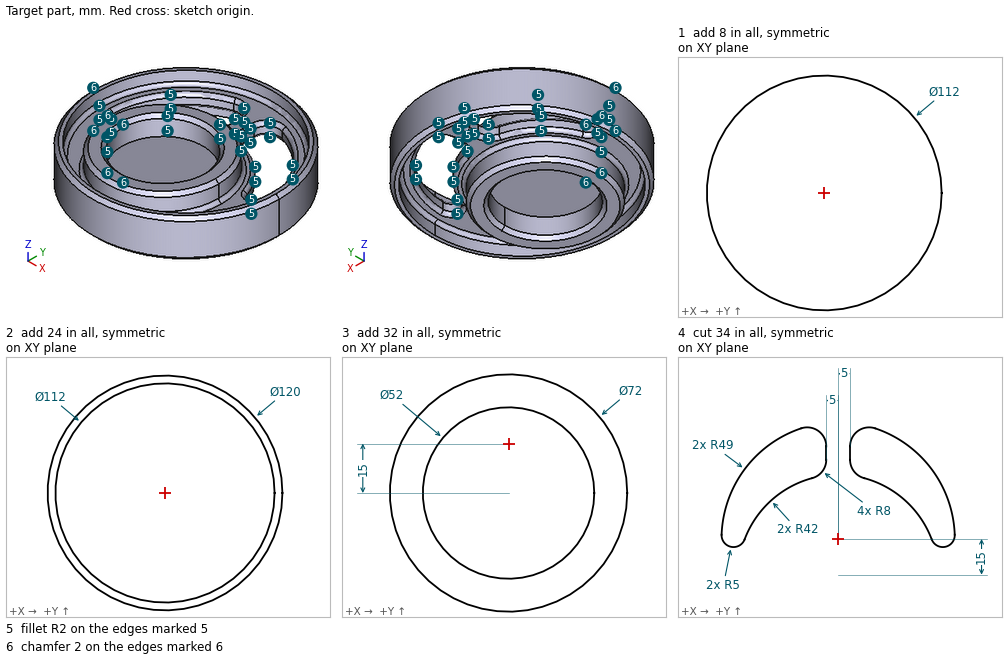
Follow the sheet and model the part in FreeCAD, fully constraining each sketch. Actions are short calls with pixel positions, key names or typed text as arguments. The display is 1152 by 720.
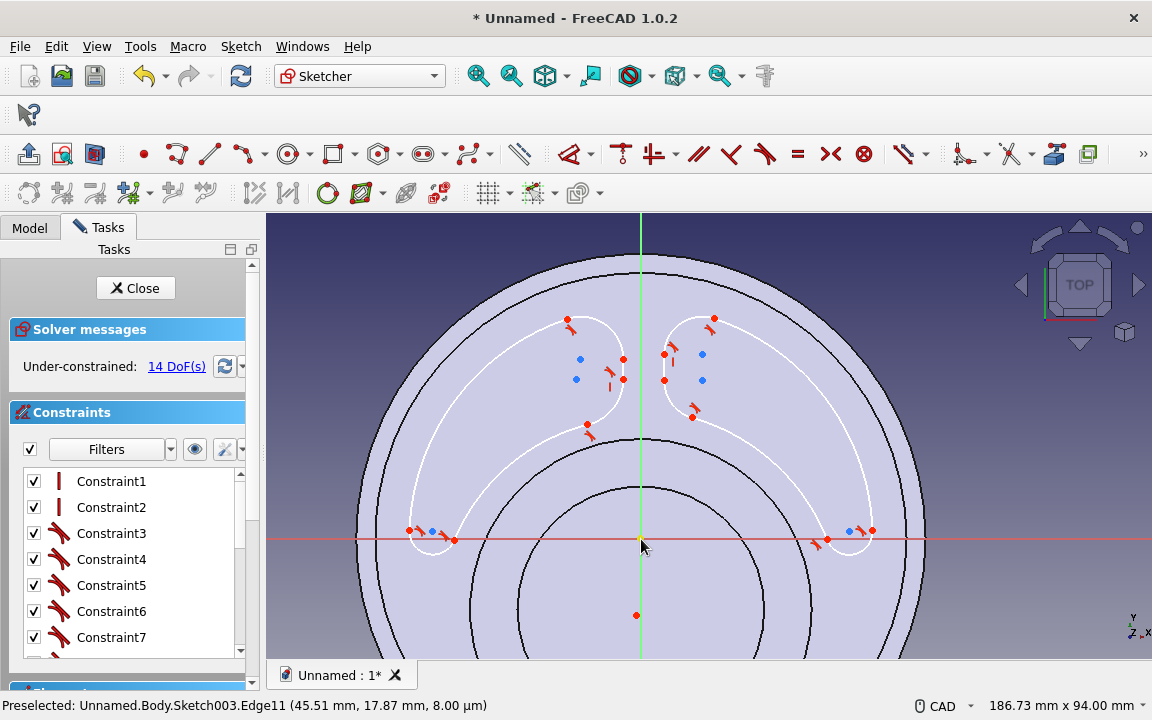
click(617, 336)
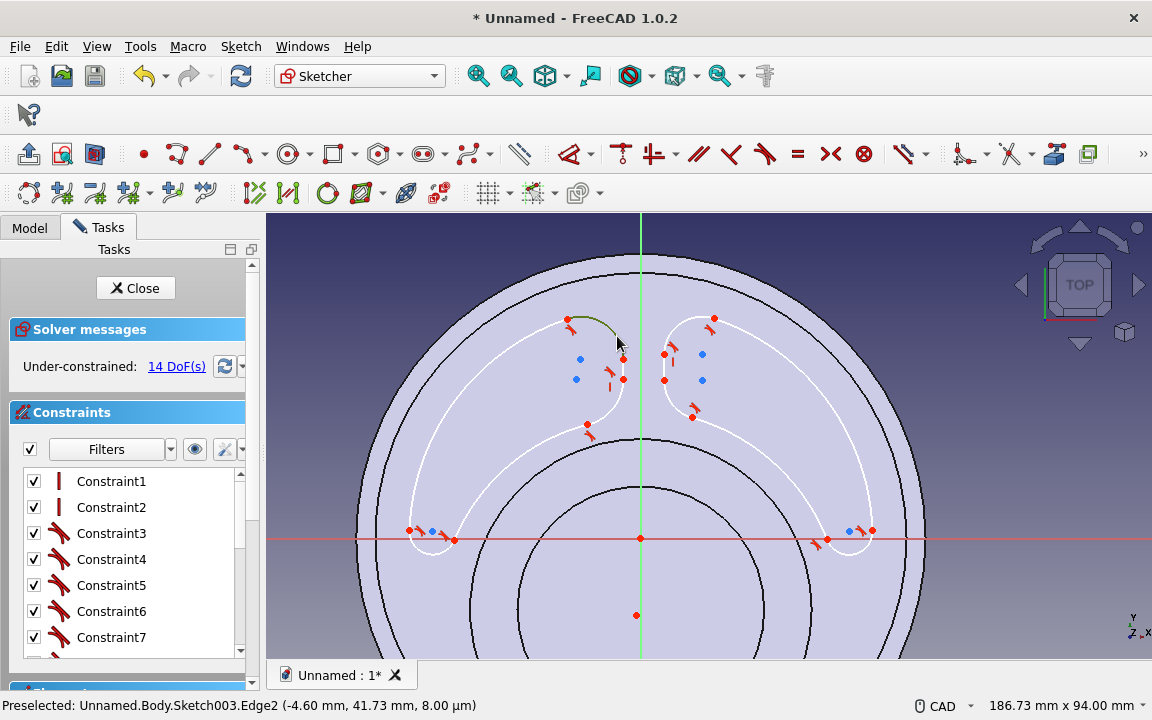
click(605, 417)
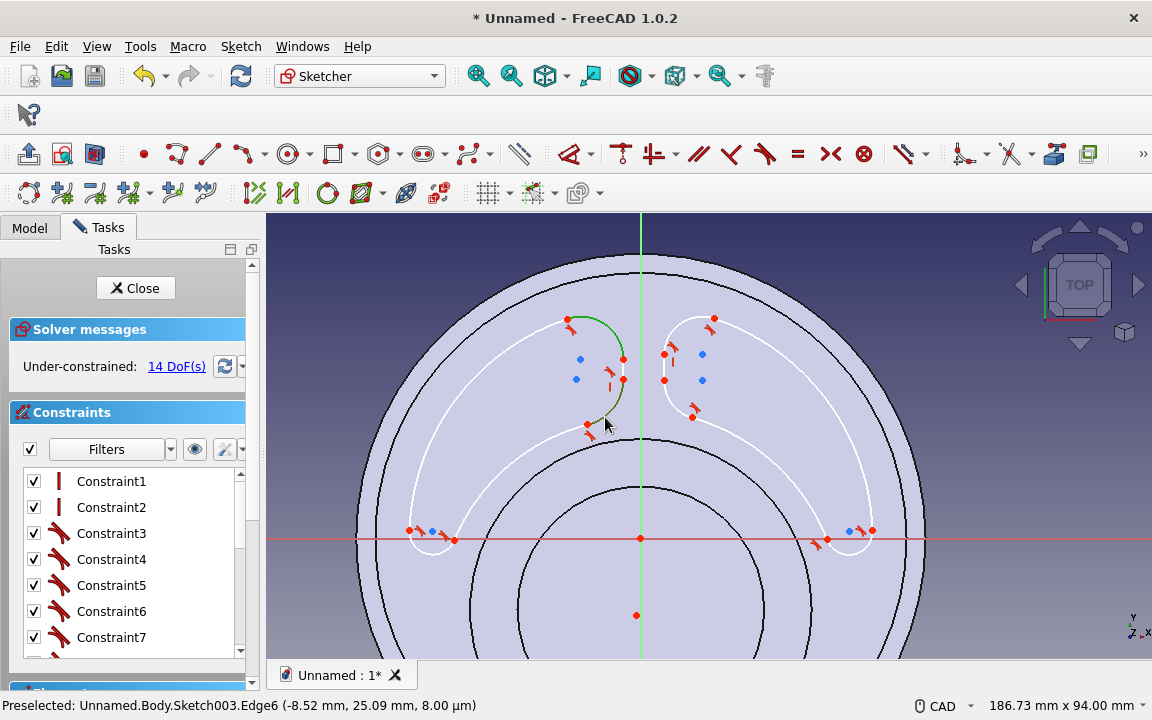
click(667, 395)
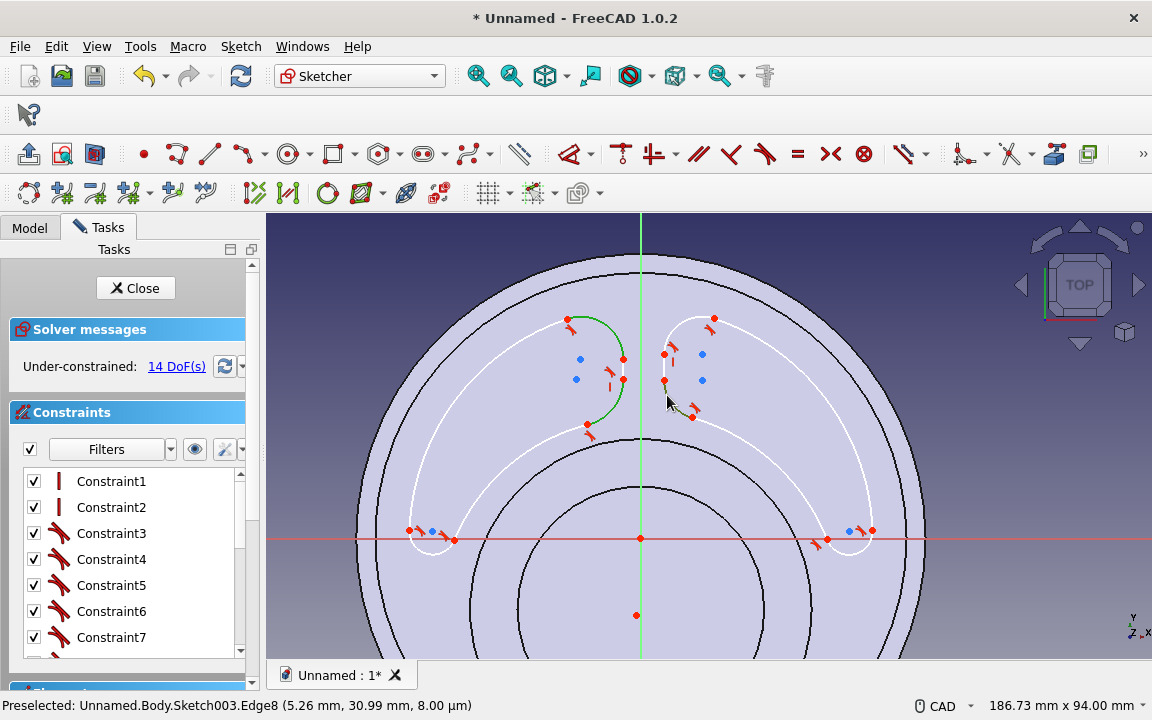
click(693, 318)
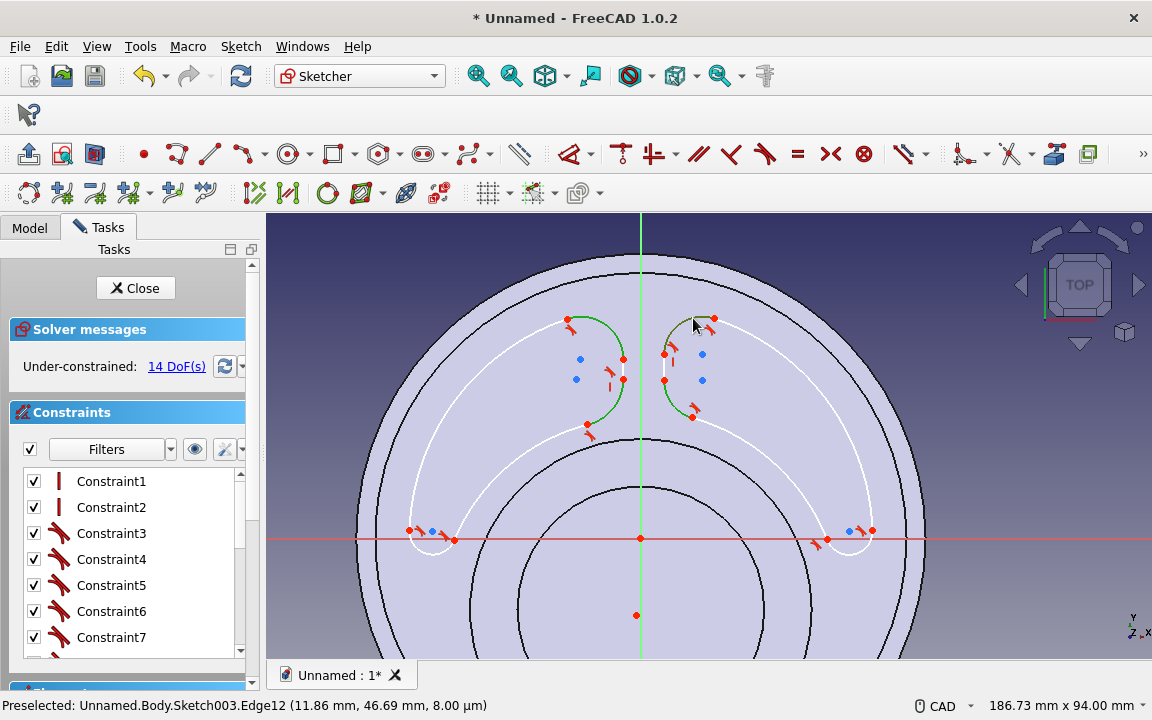
key(e)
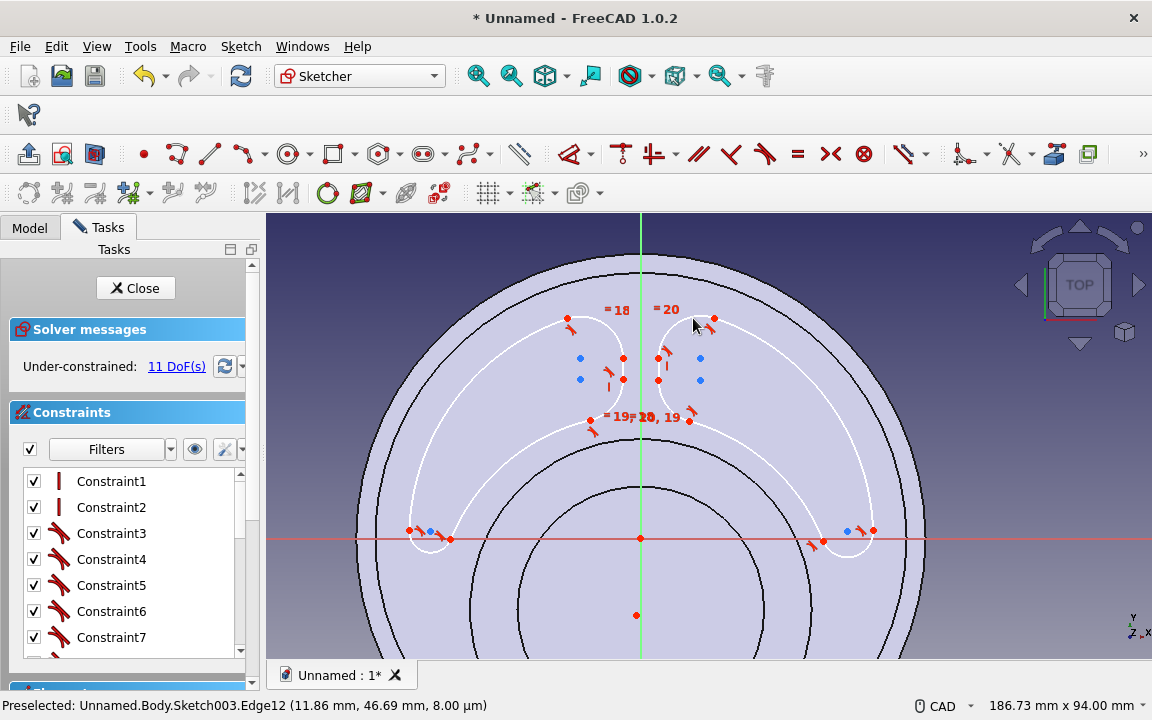
click(537, 441)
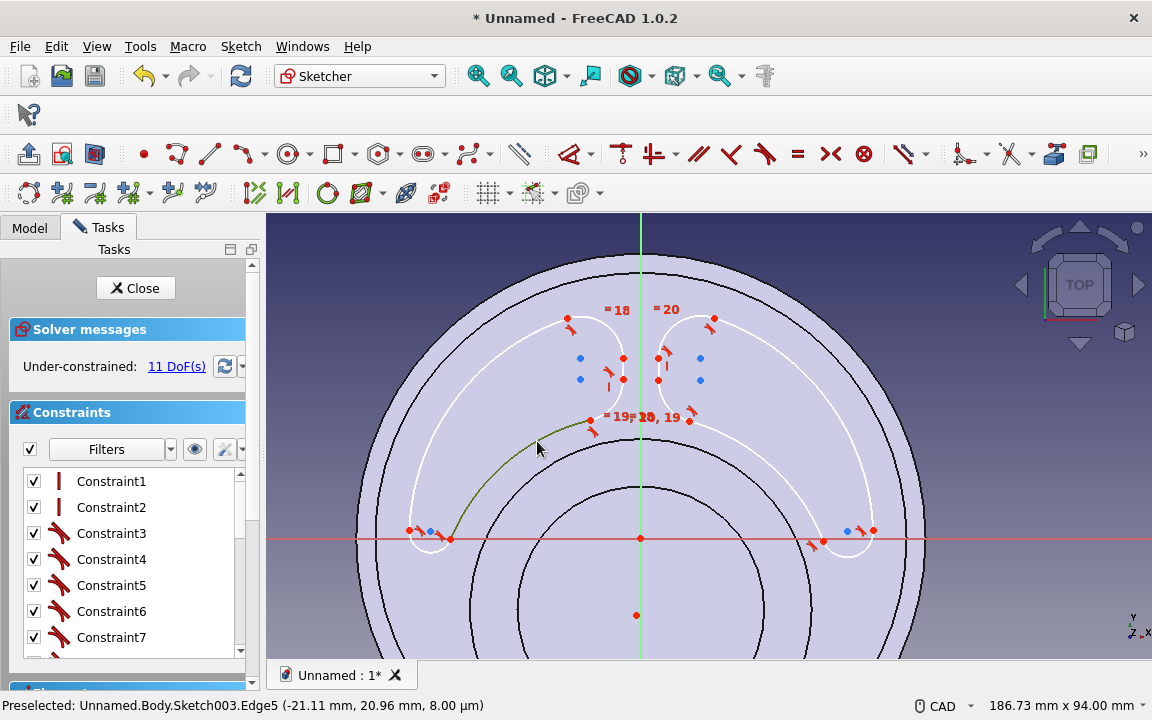
click(796, 493)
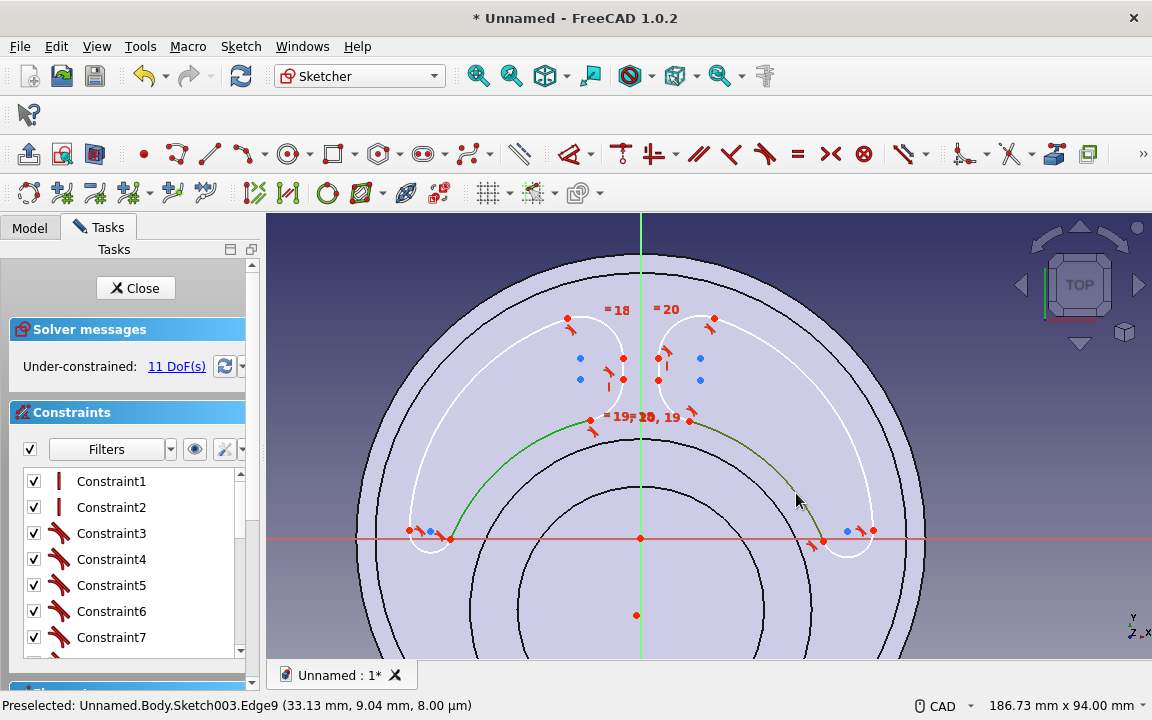
key(e)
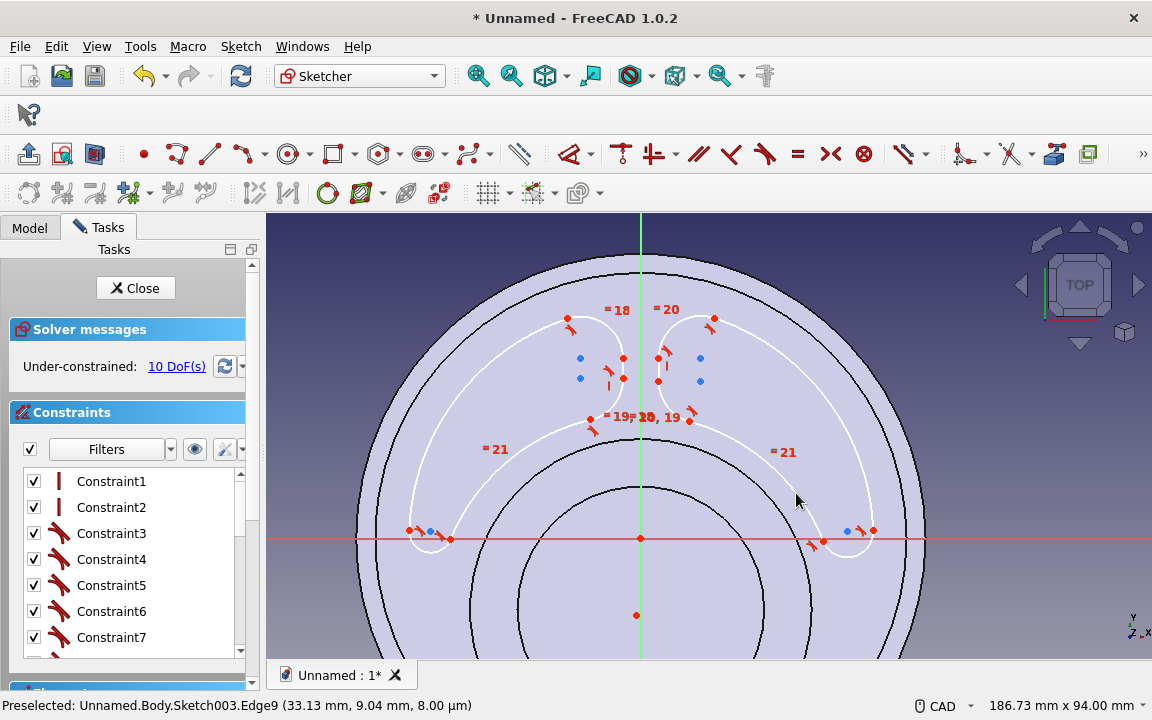
click(438, 551)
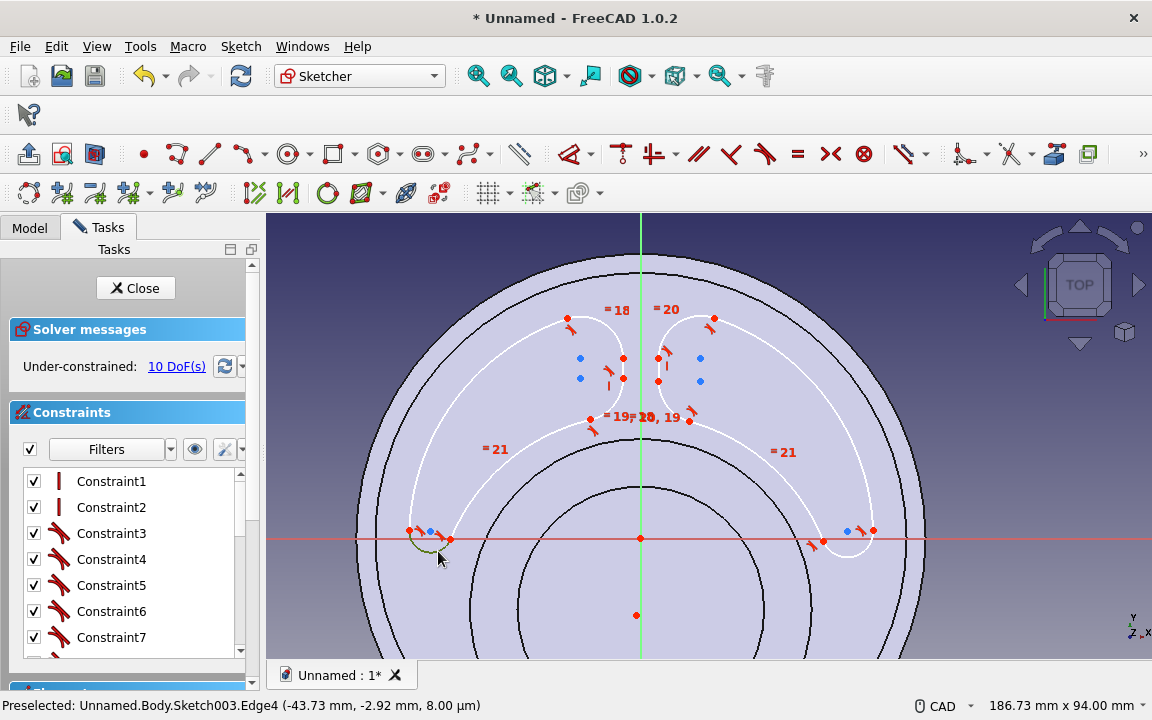
click(838, 556)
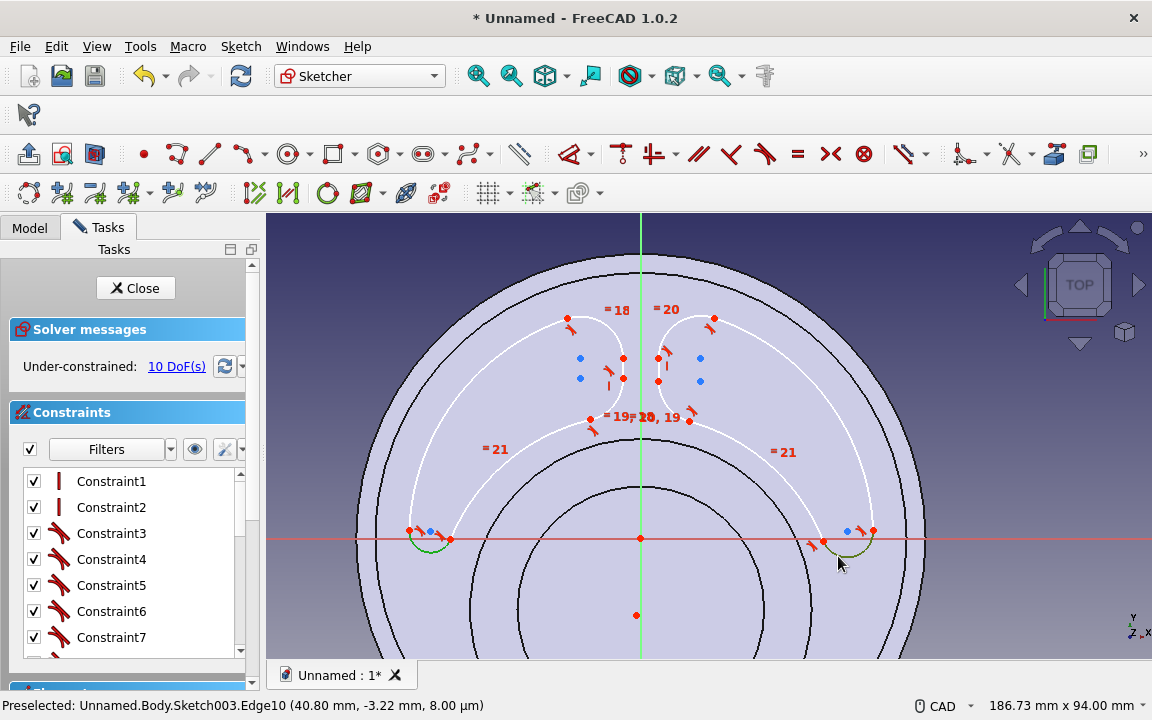
click(798, 154)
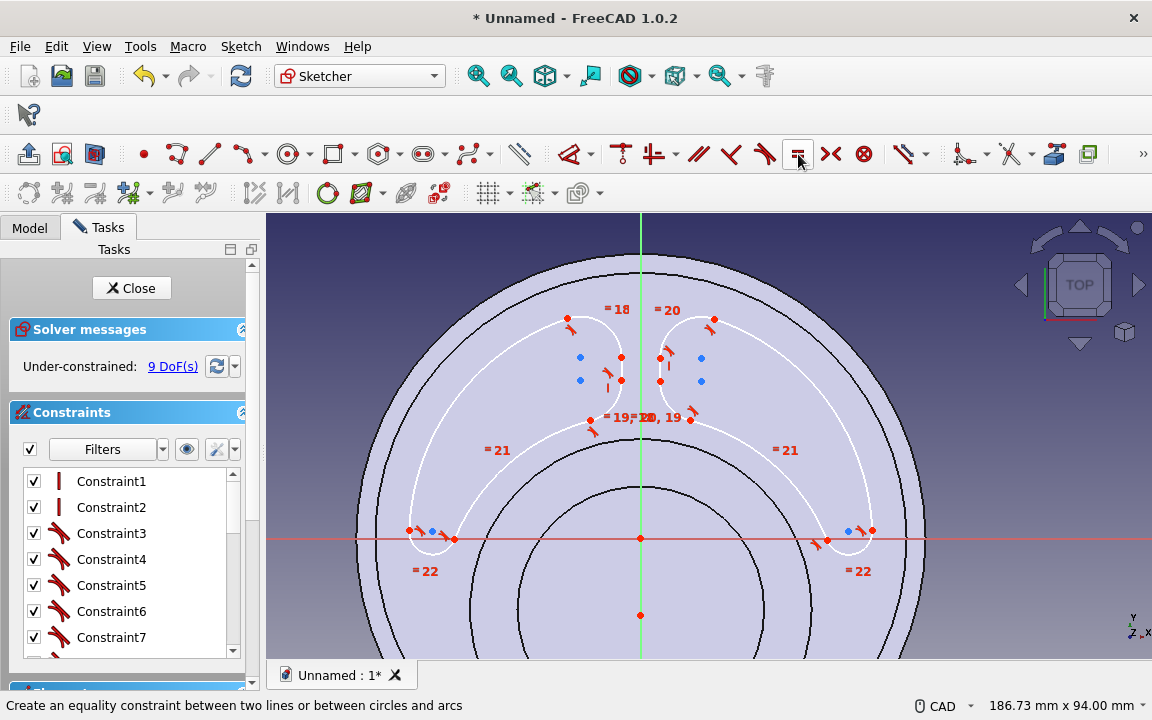
click(494, 359)